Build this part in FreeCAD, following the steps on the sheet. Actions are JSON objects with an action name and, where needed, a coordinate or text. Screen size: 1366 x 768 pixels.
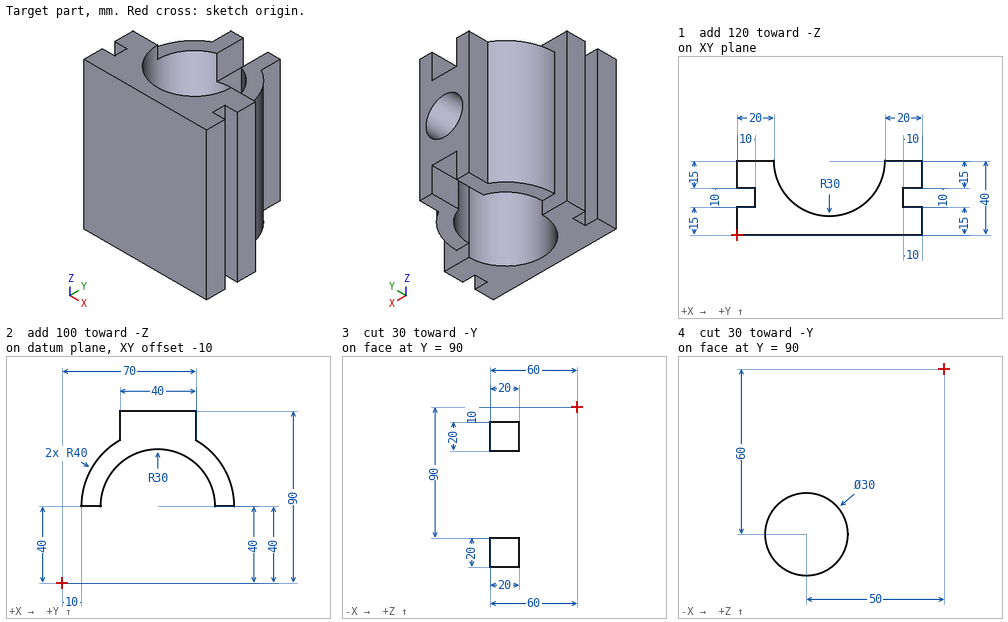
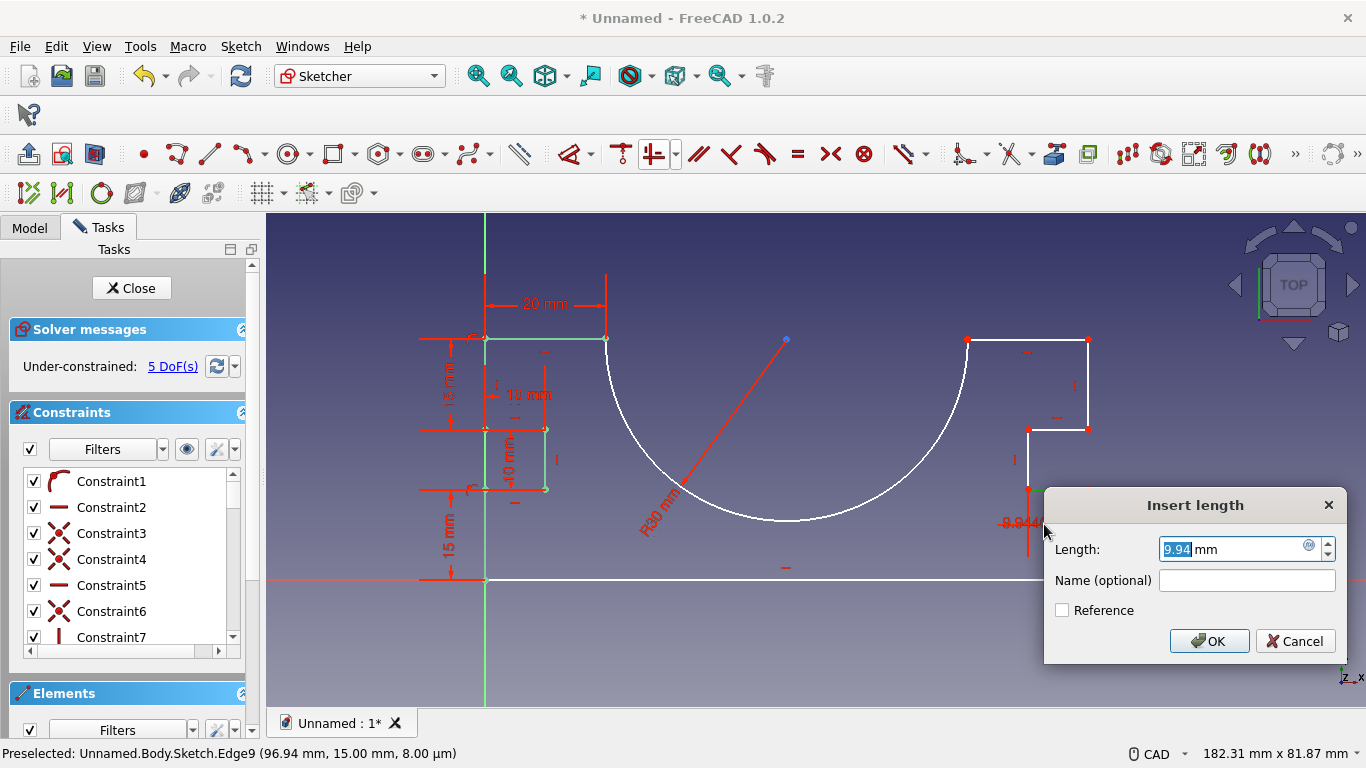
{"action": "type", "text": "10"}
{"action": "key", "text": "Return"}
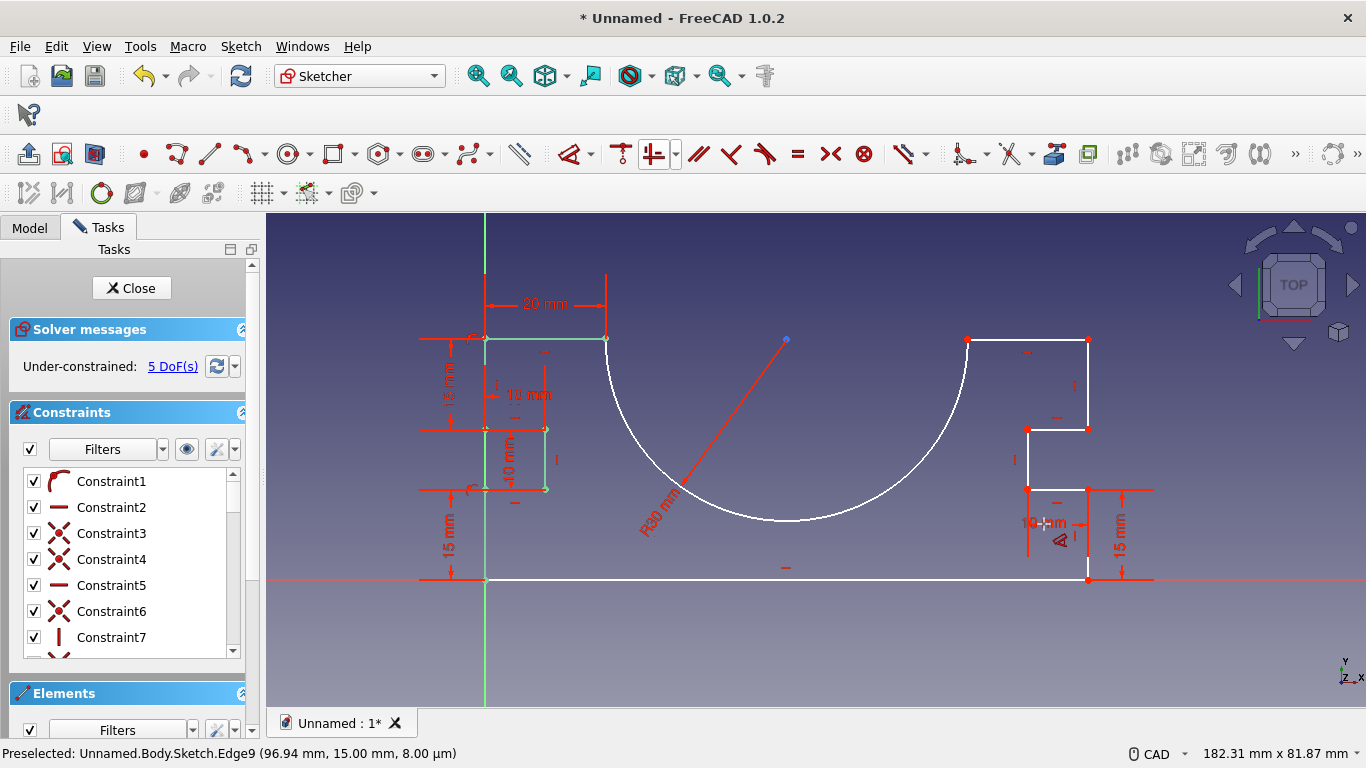
{"action": "left_click", "coordinate": [1028, 472]}
{"action": "left_click", "coordinate": [1062, 460]}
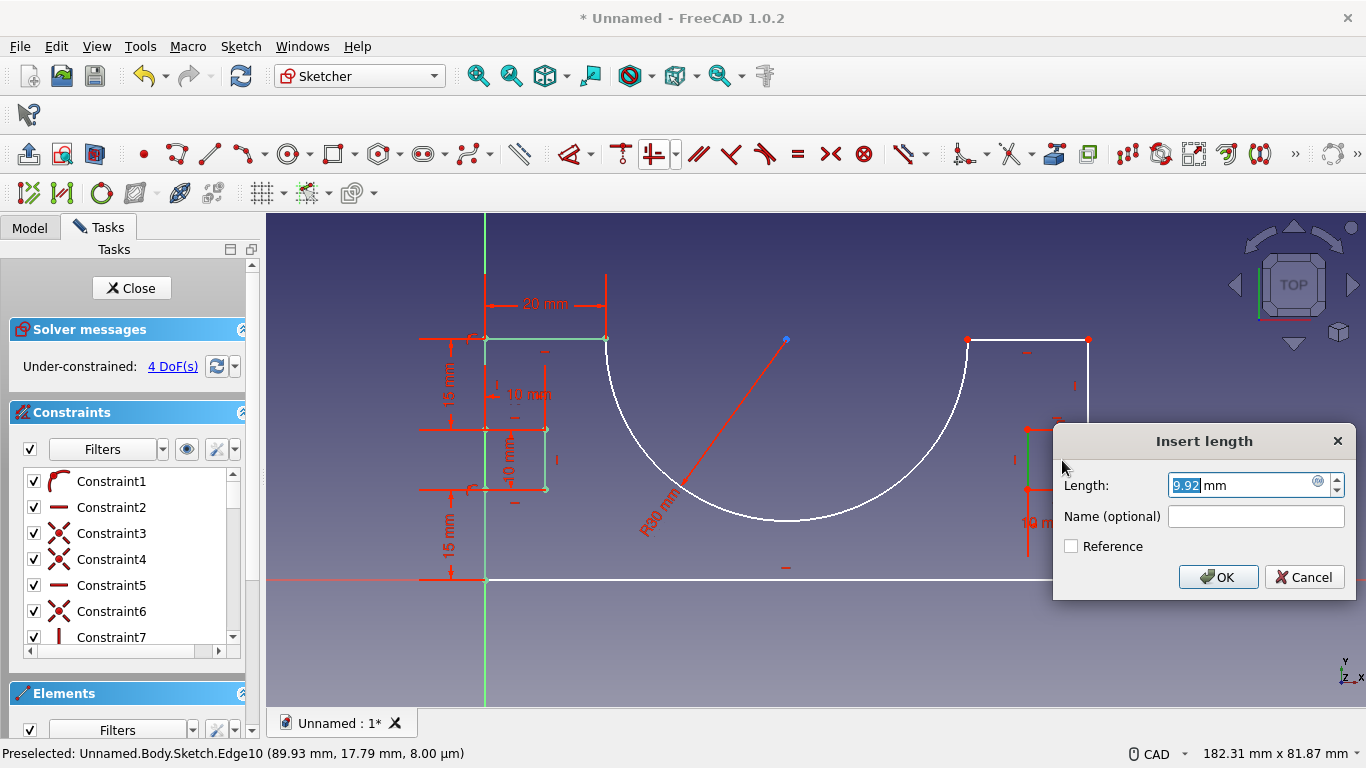
{"action": "type", "text": "10"}
{"action": "key", "text": "Return"}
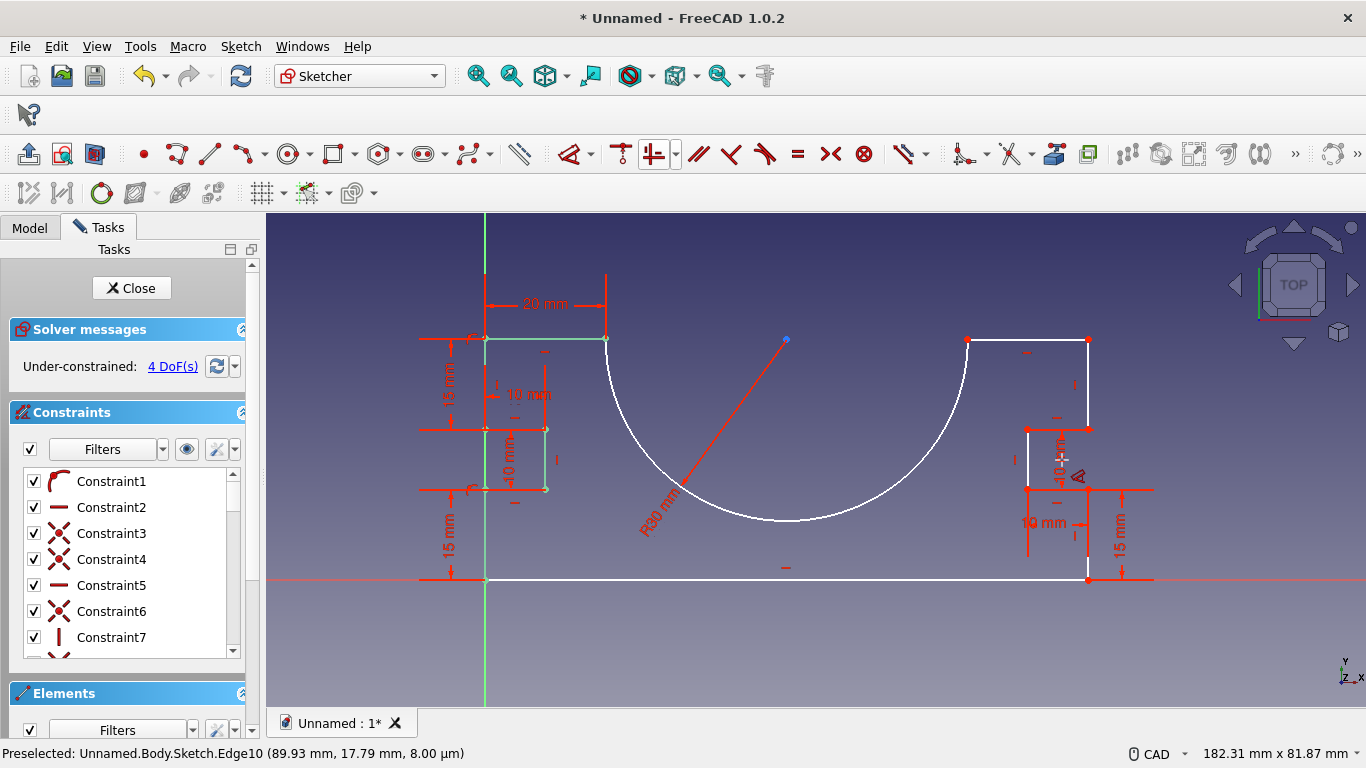
{"action": "left_click", "coordinate": [1046, 429]}
{"action": "left_click", "coordinate": [1058, 395]}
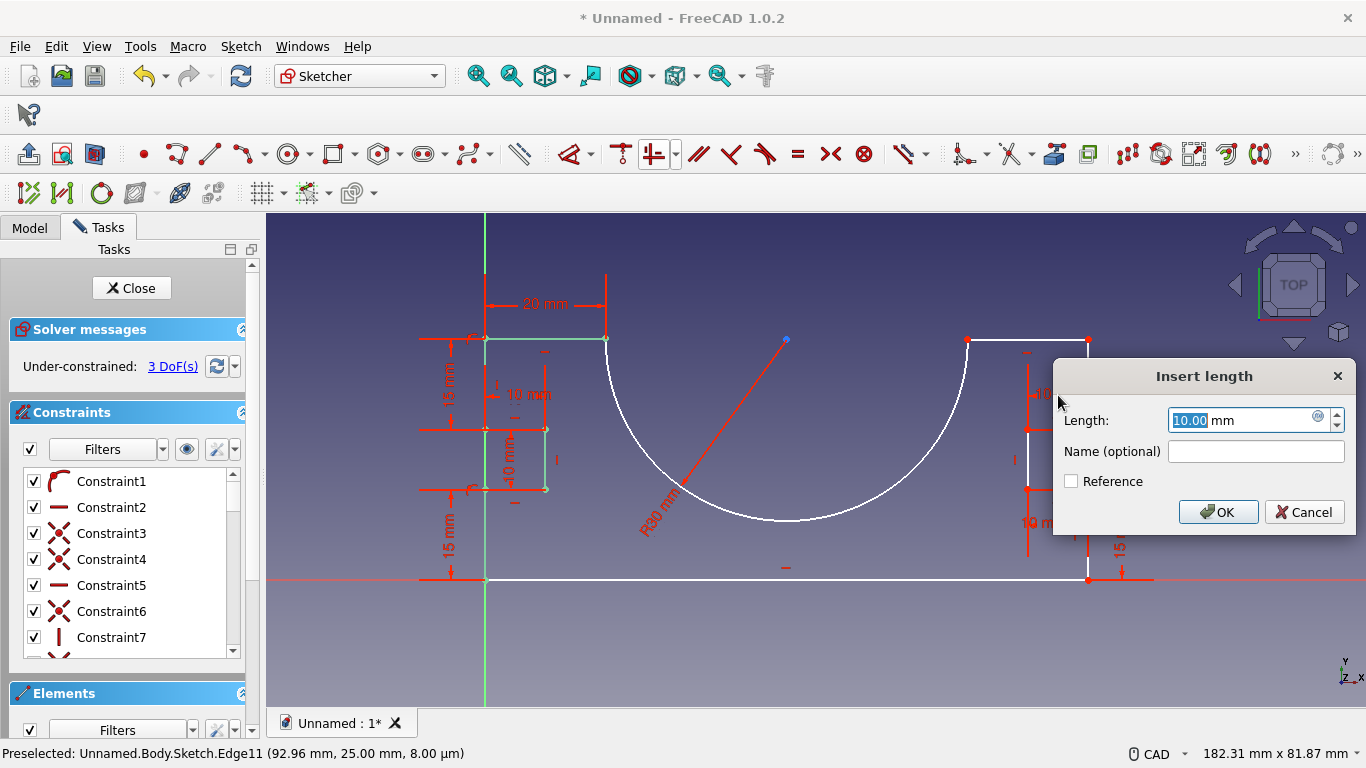
{"action": "type", "text": "10"}
{"action": "key", "text": "Return"}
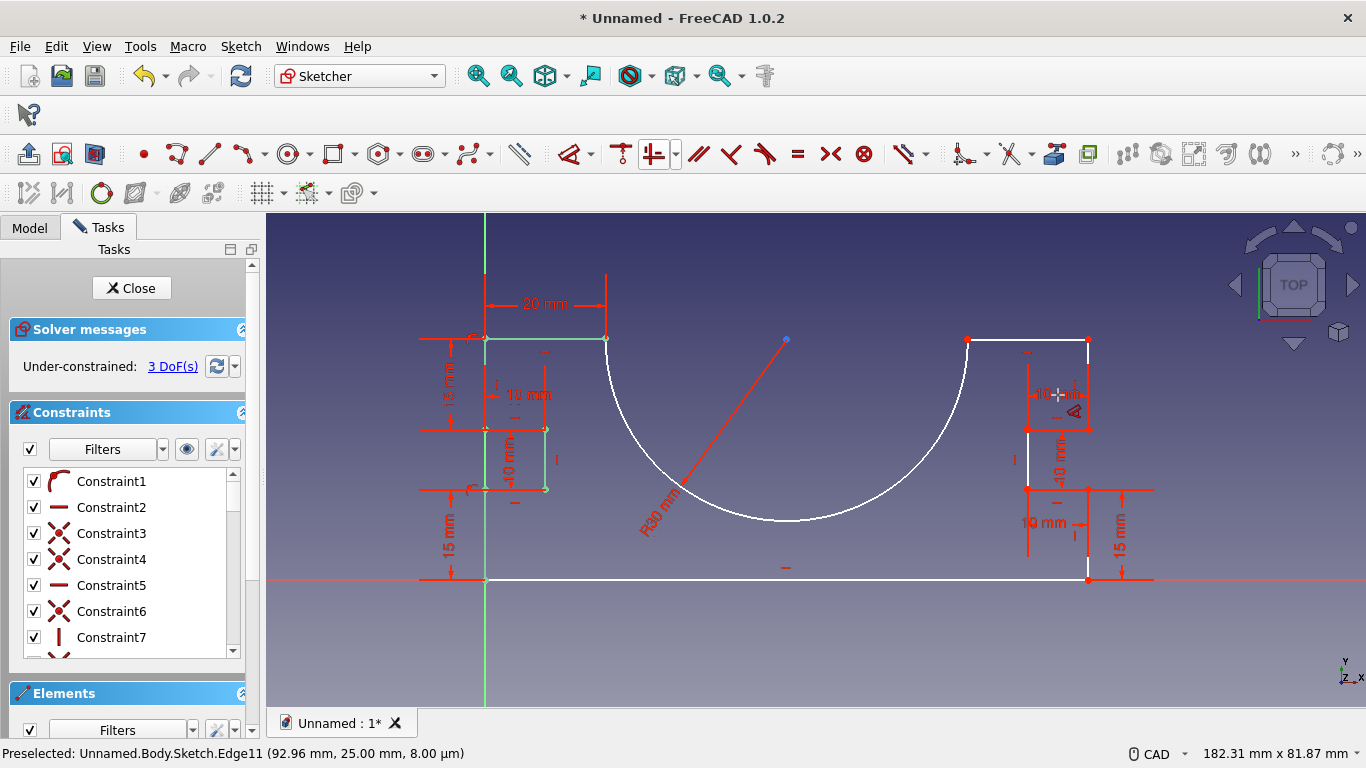
{"action": "left_click", "coordinate": [1088, 403]}
{"action": "left_click", "coordinate": [1122, 364]}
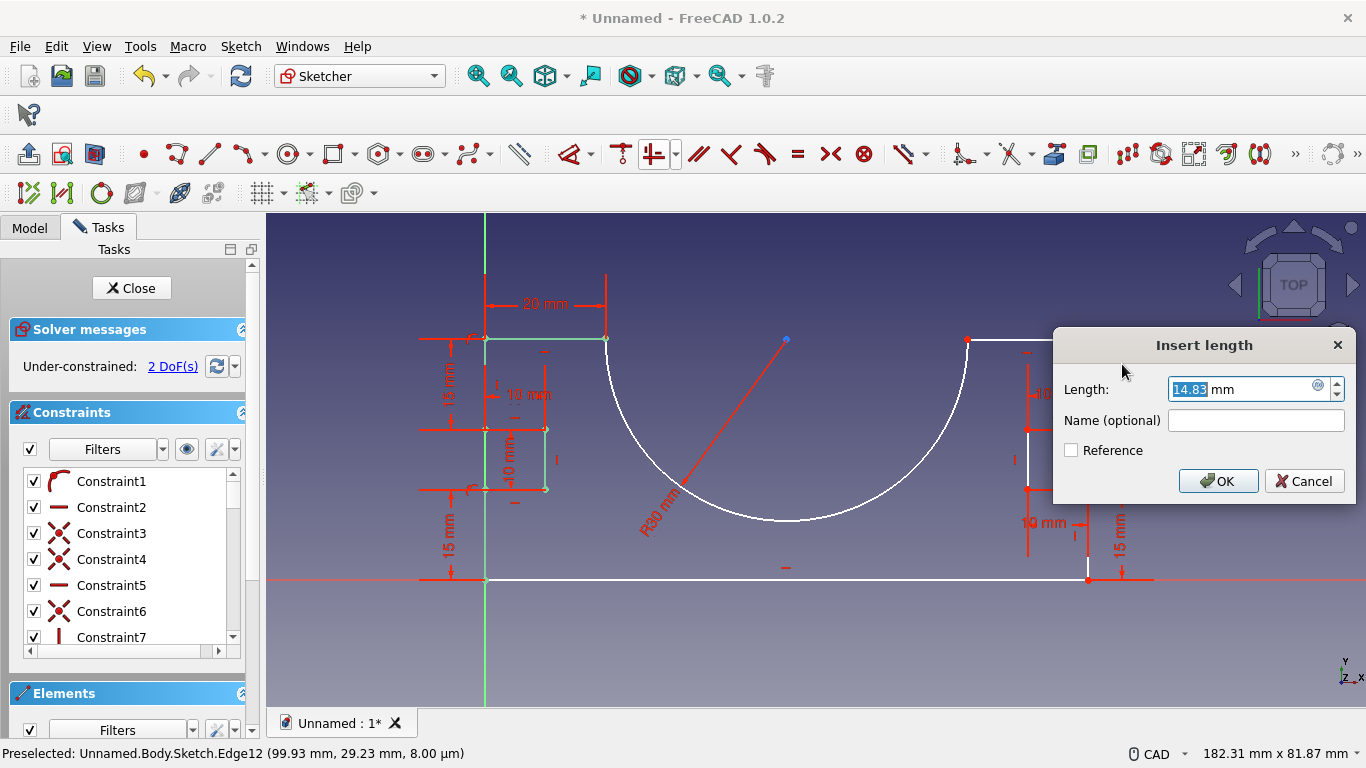
{"action": "type", "text": "15"}
{"action": "key", "text": "Return"}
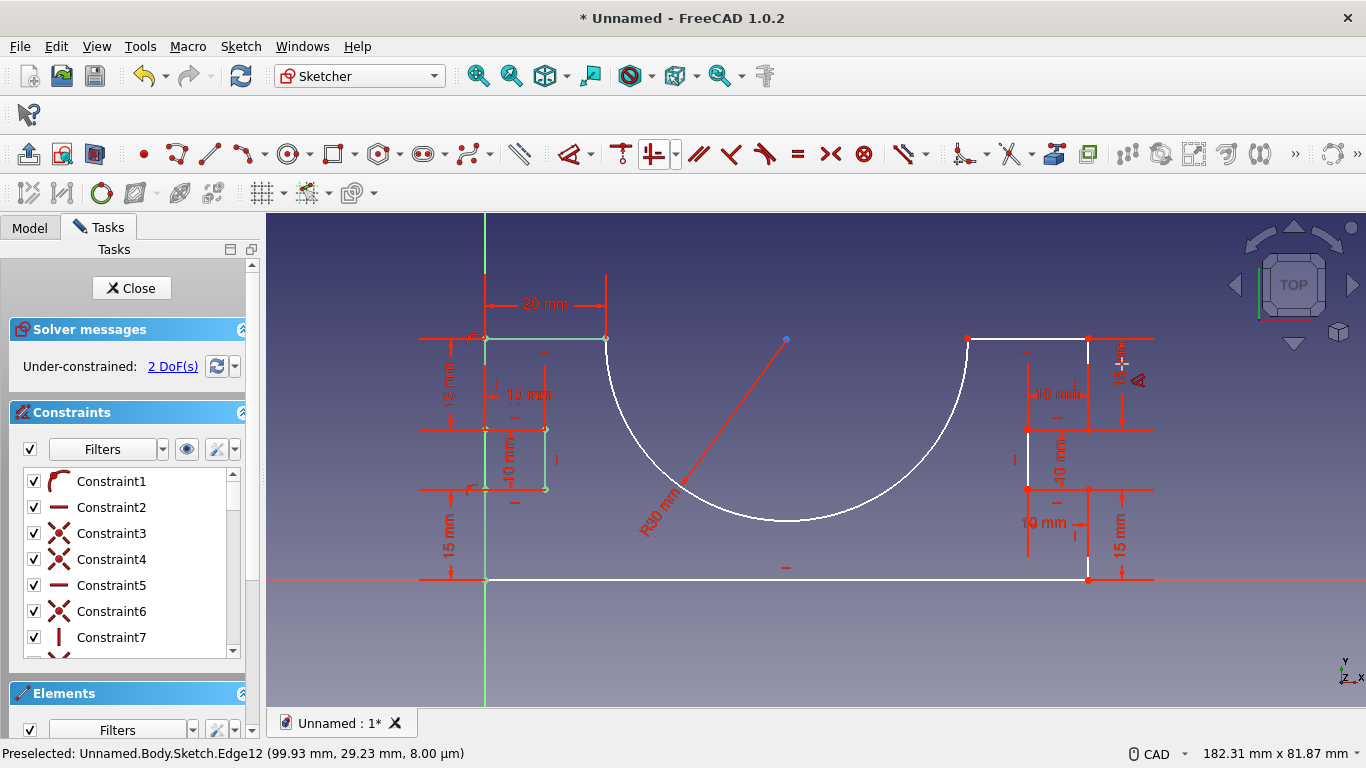
{"action": "left_click", "coordinate": [1052, 339]}
{"action": "left_click", "coordinate": [1028, 305]}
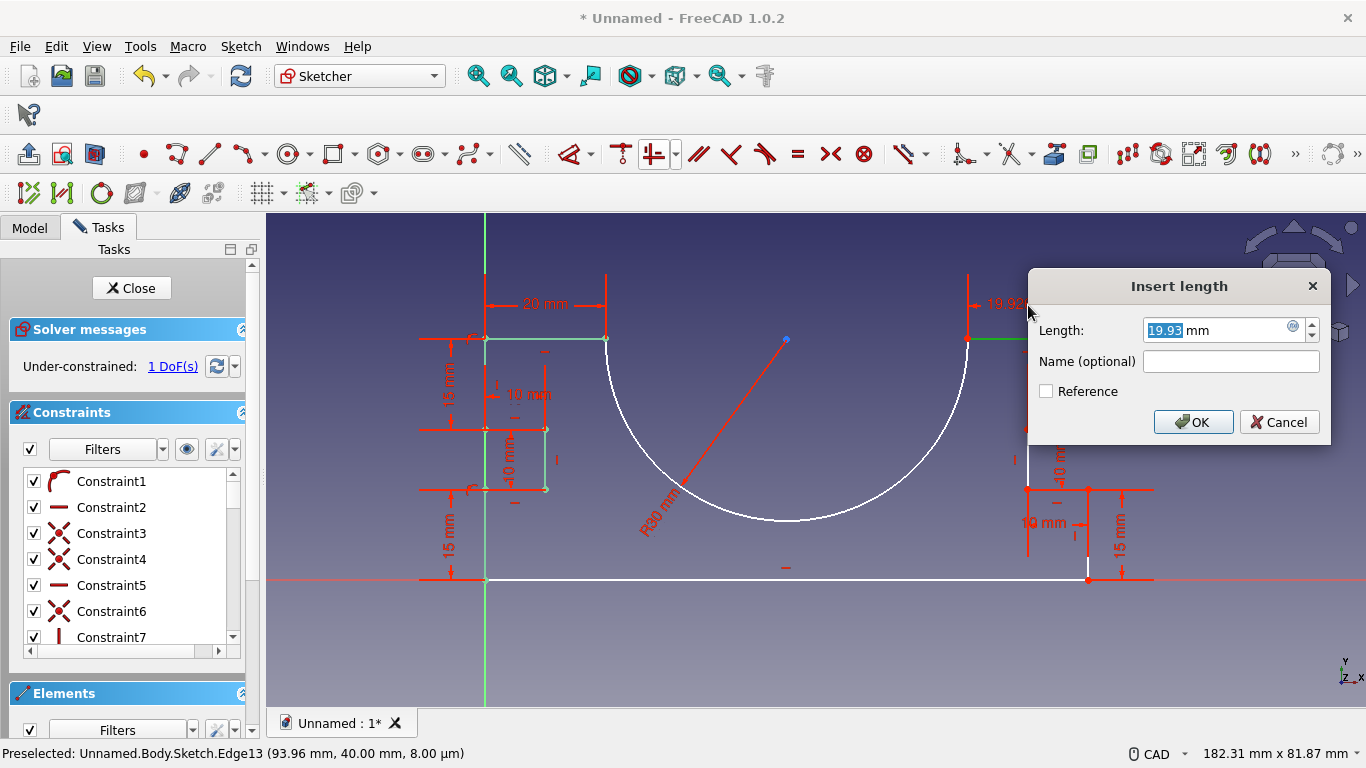
{"action": "type", "text": "20"}
{"action": "key", "text": "Return"}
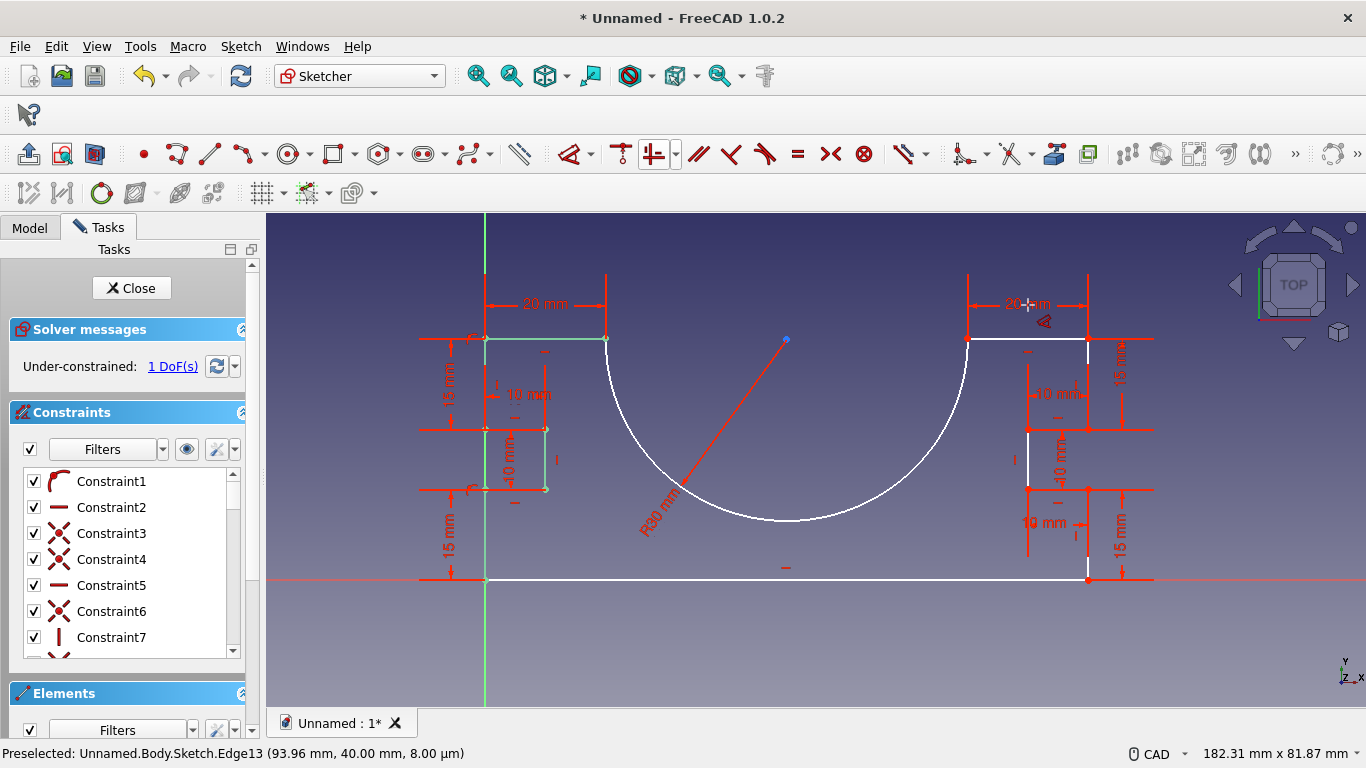
{"action": "left_click", "coordinate": [787, 340]}
{"action": "left_click", "coordinate": [451, 515]}